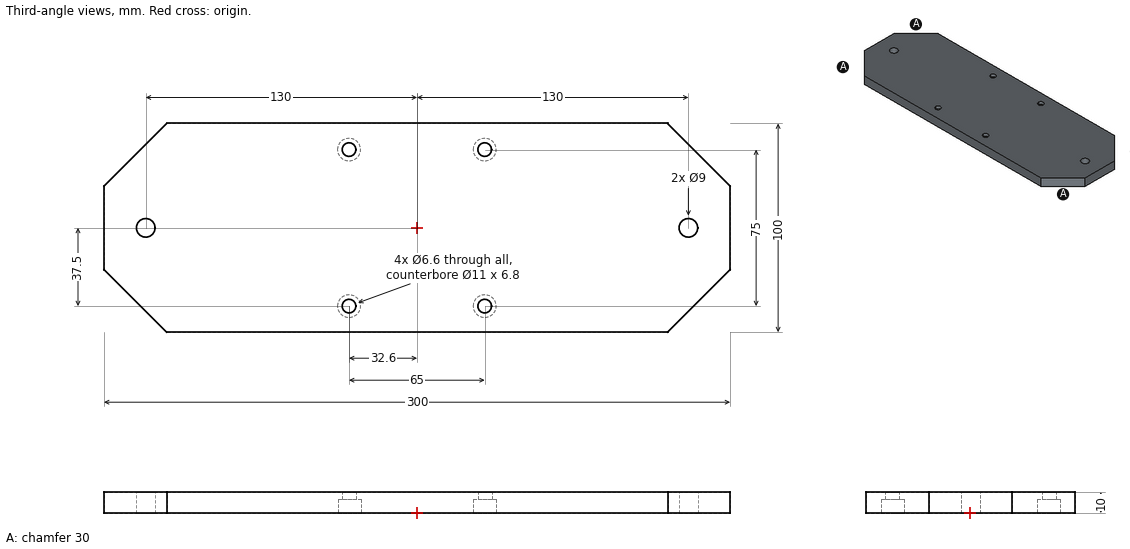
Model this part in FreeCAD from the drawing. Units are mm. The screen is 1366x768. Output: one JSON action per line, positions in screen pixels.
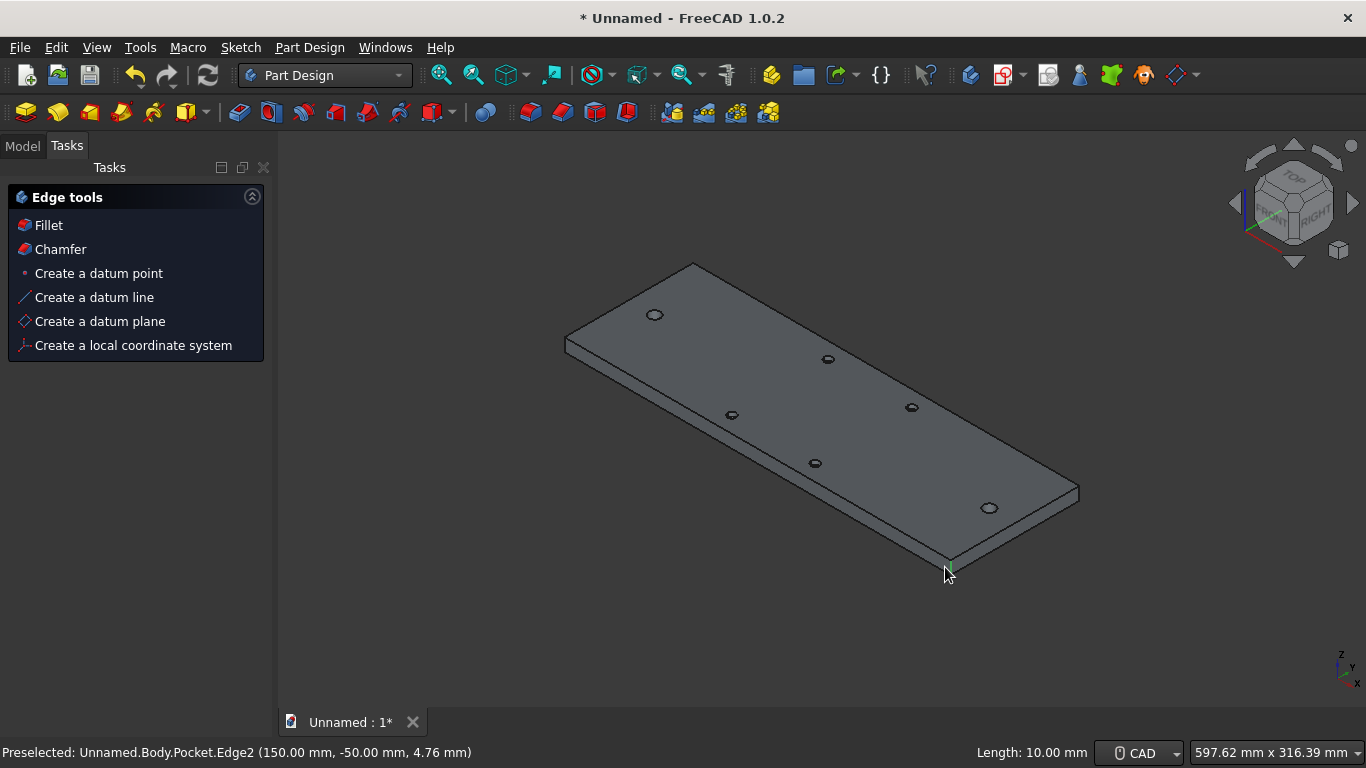
{"action": "scroll", "coordinate": [693, 269], "scroll_direction": "up", "scroll_amount": 4}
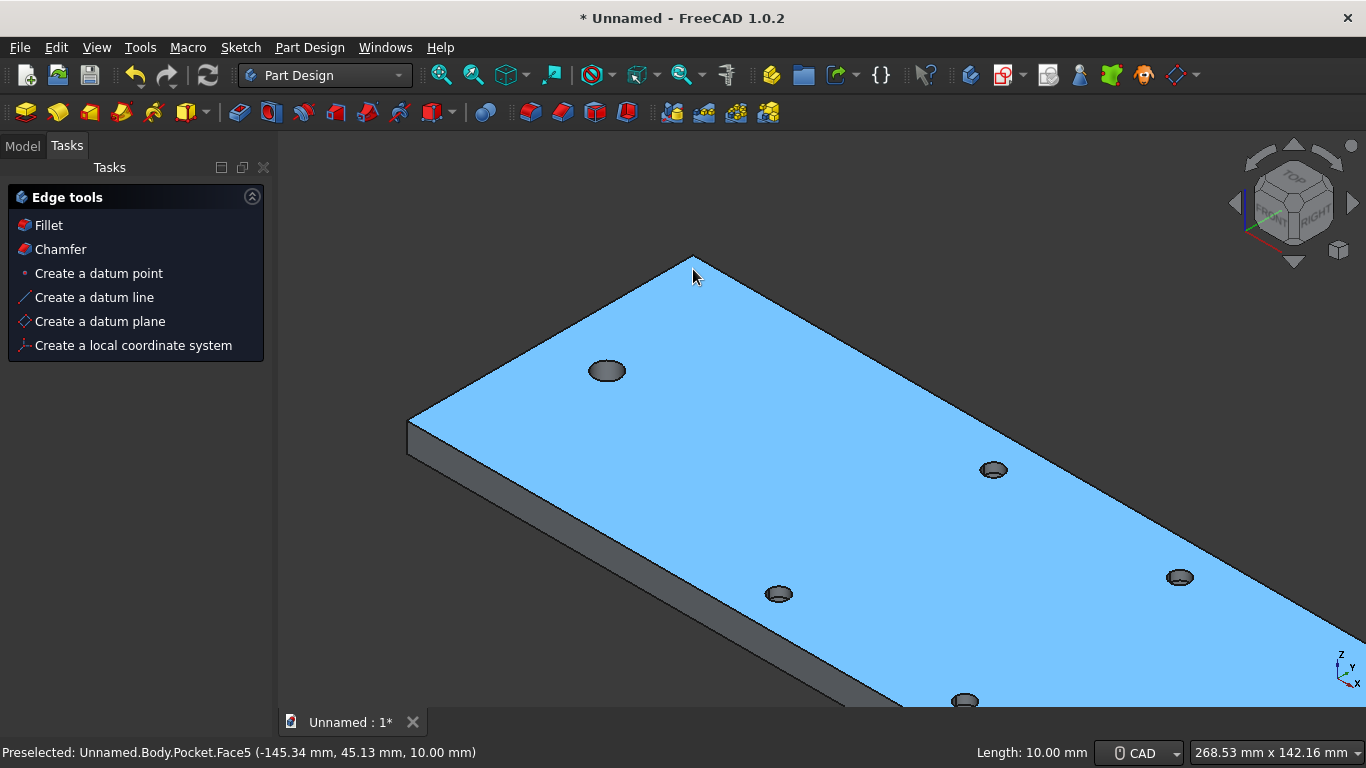
{"action": "left_click", "coordinate": [442, 76]}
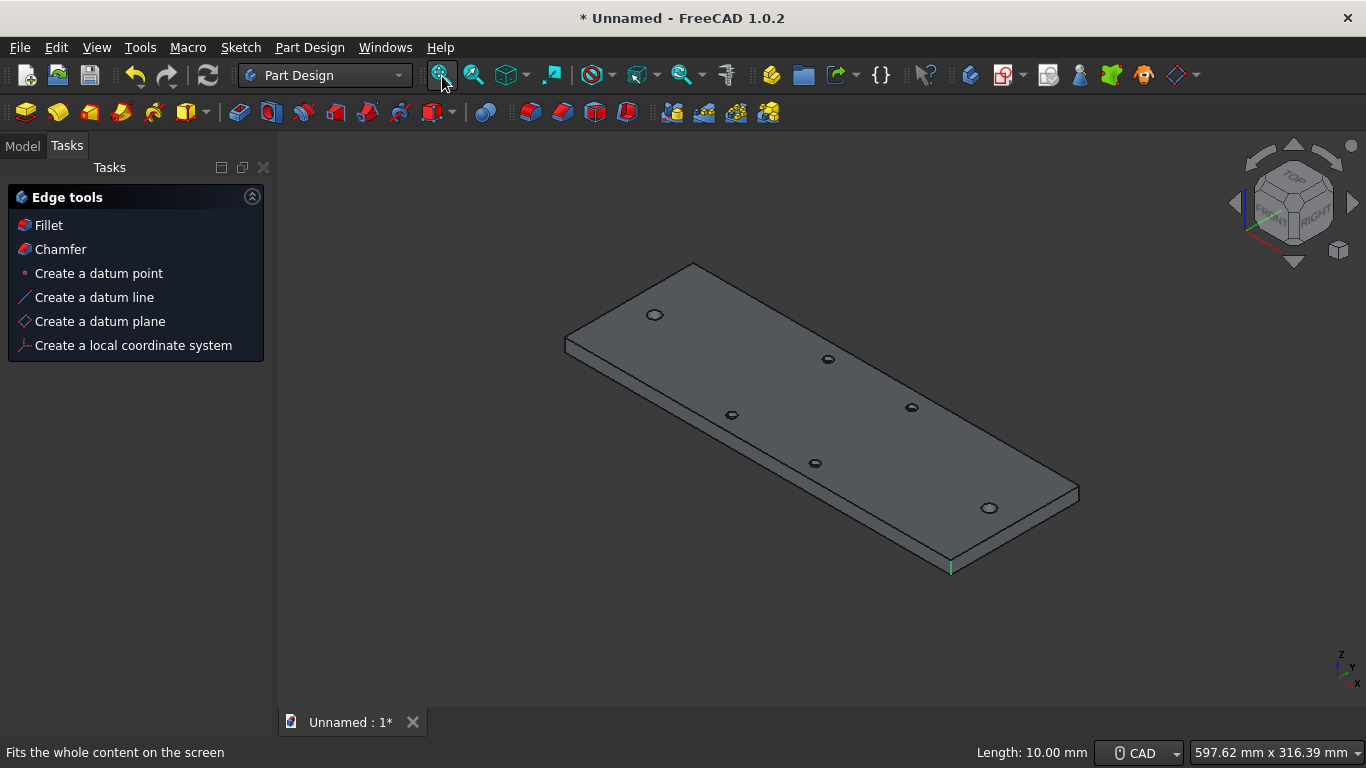
{"action": "key", "text": "2"}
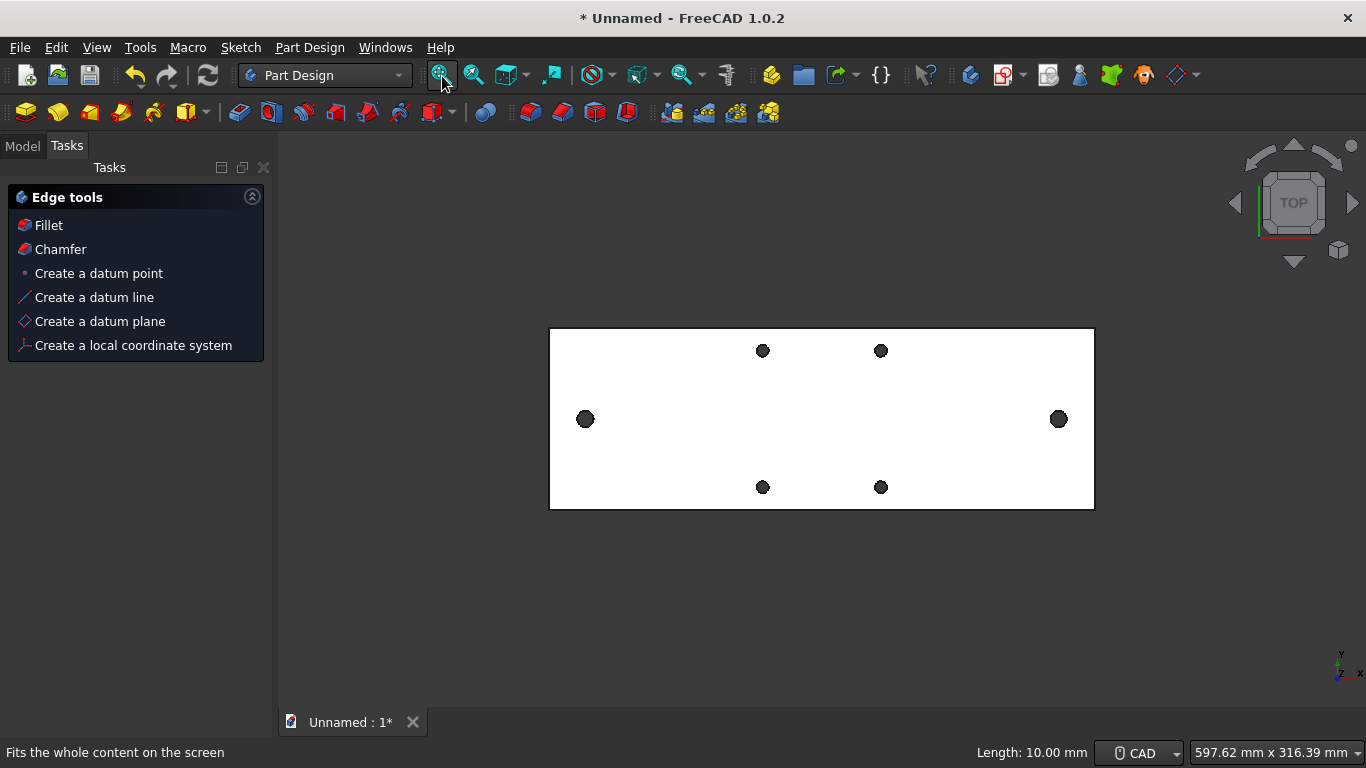
{"action": "scroll", "coordinate": [549, 327], "scroll_direction": "up", "scroll_amount": 4}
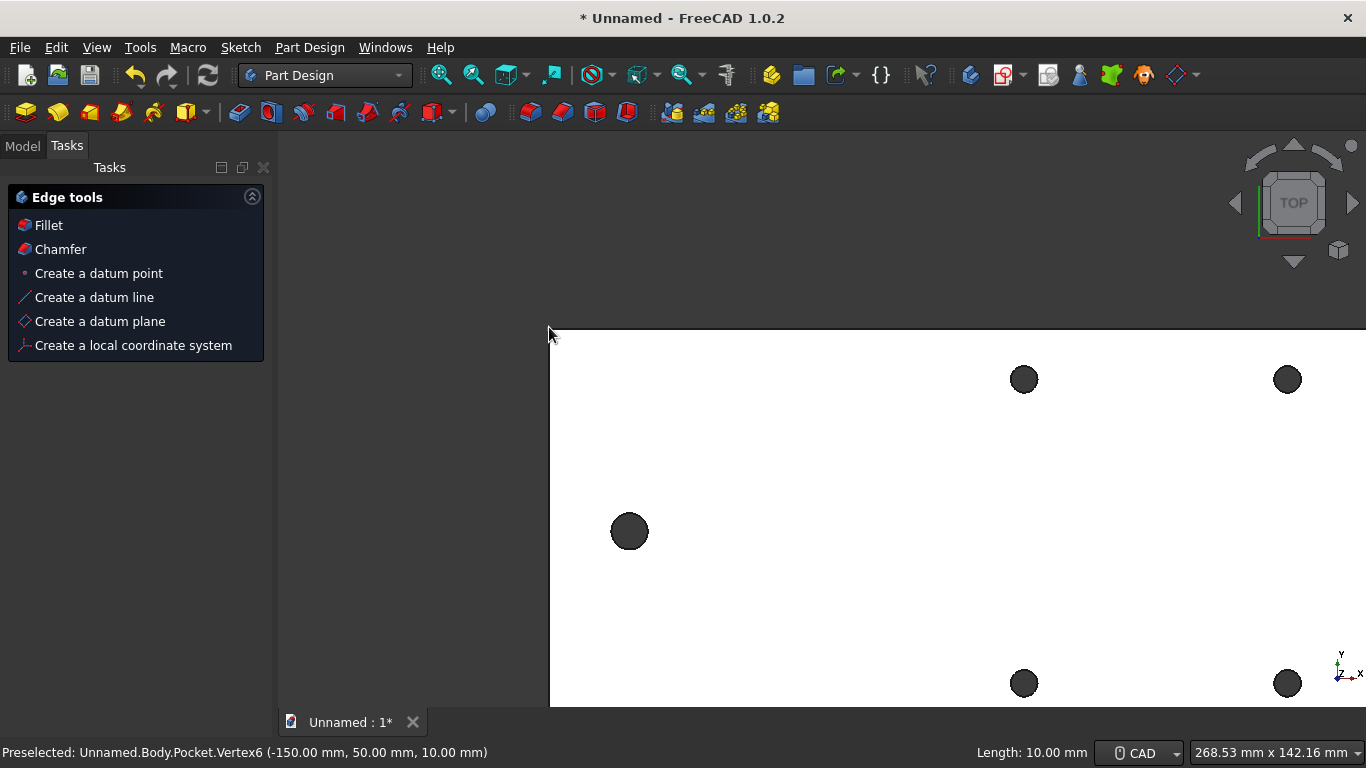
{"action": "key", "text": "v f"}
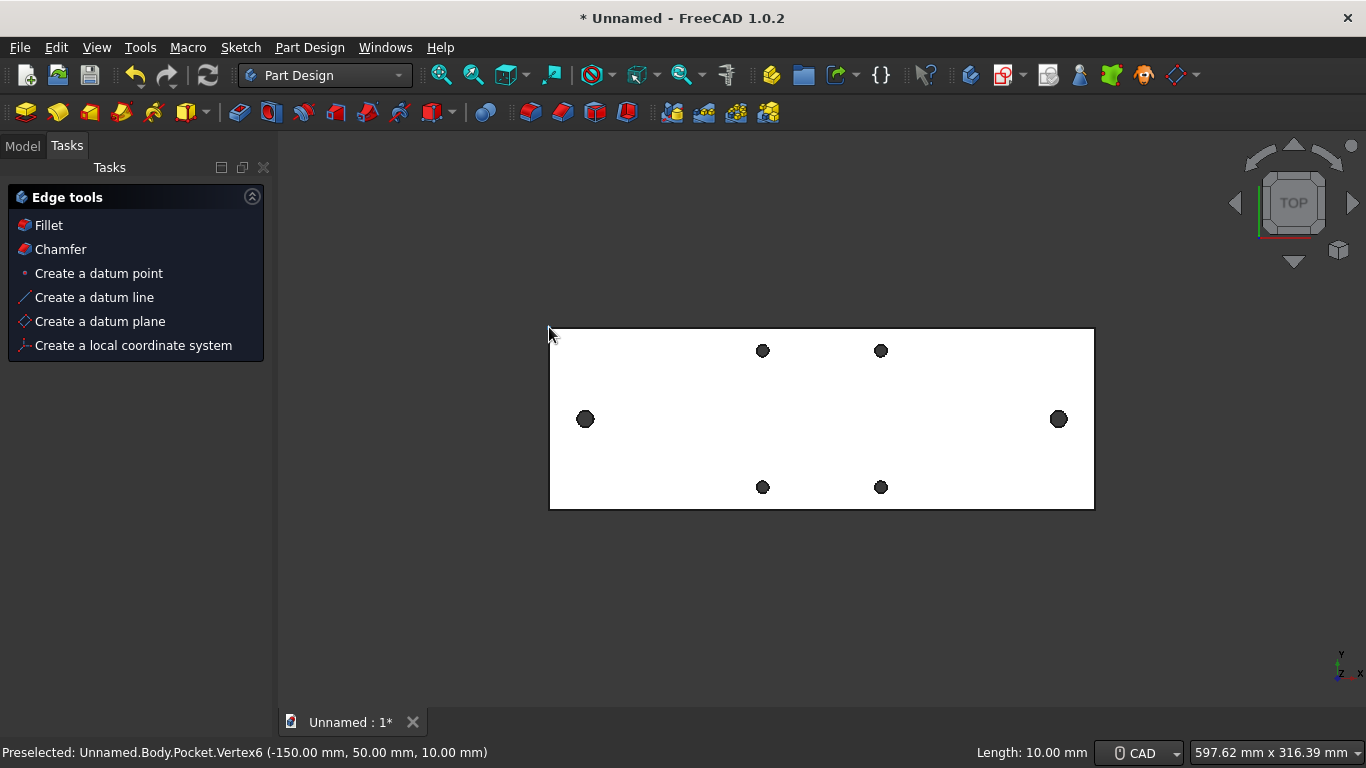
{"action": "key", "text": "1"}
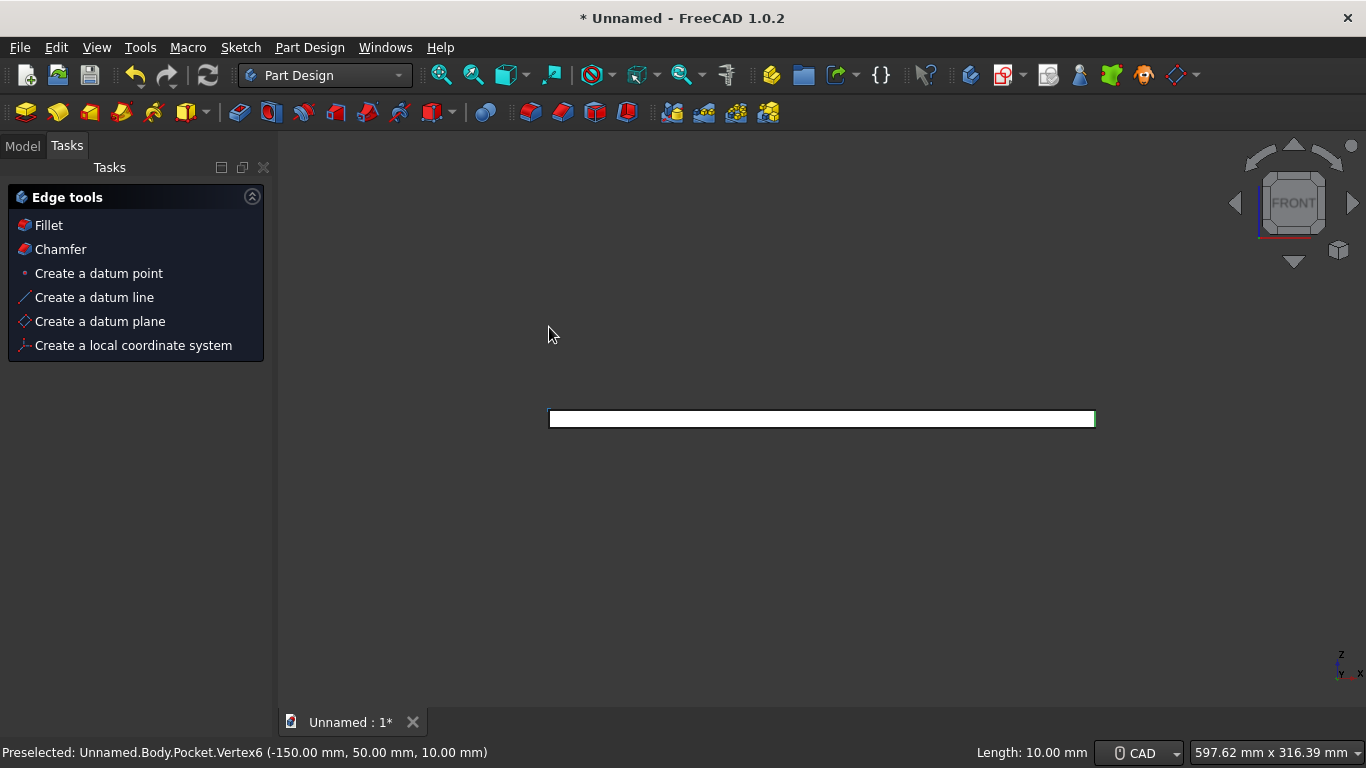
{"action": "left_click", "coordinate": [549, 418], "text": "ctrl"}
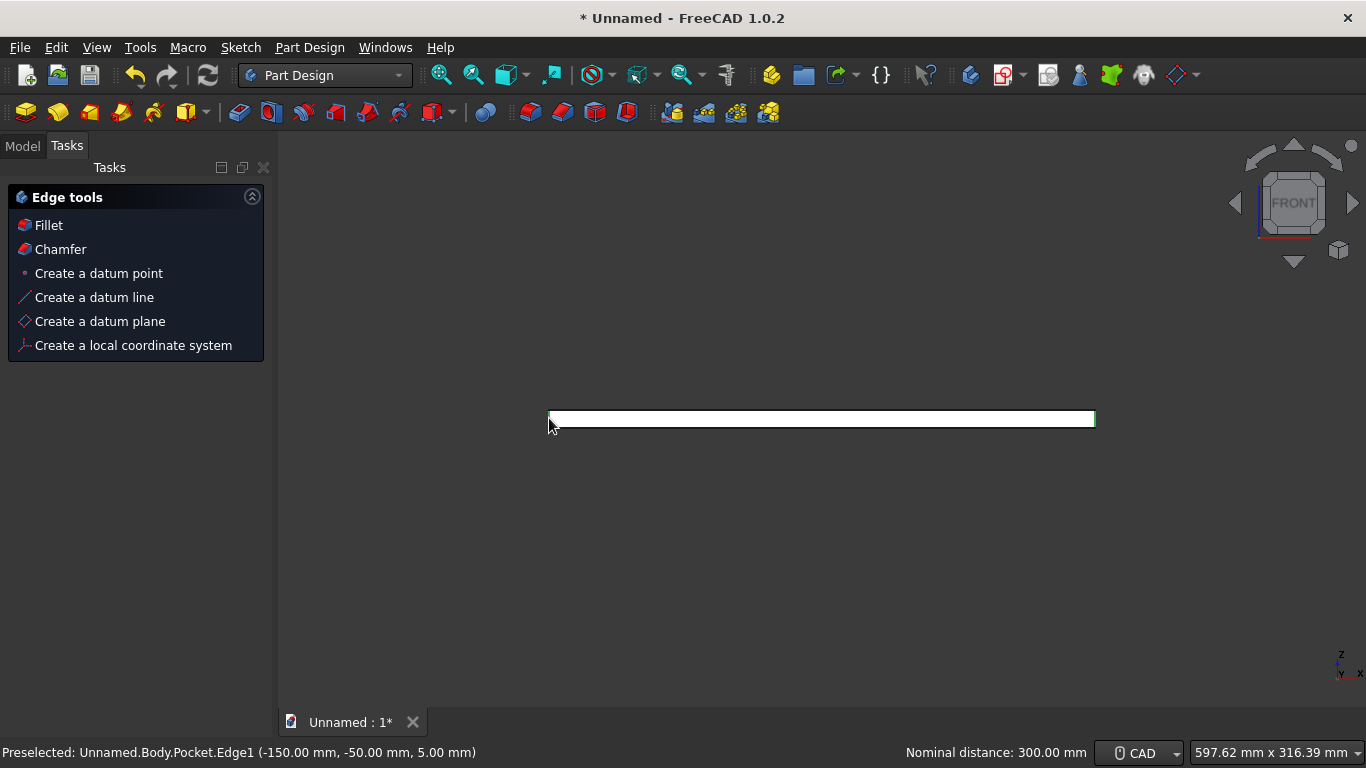
{"action": "scroll", "coordinate": [549, 418], "scroll_direction": "up", "scroll_amount": 4}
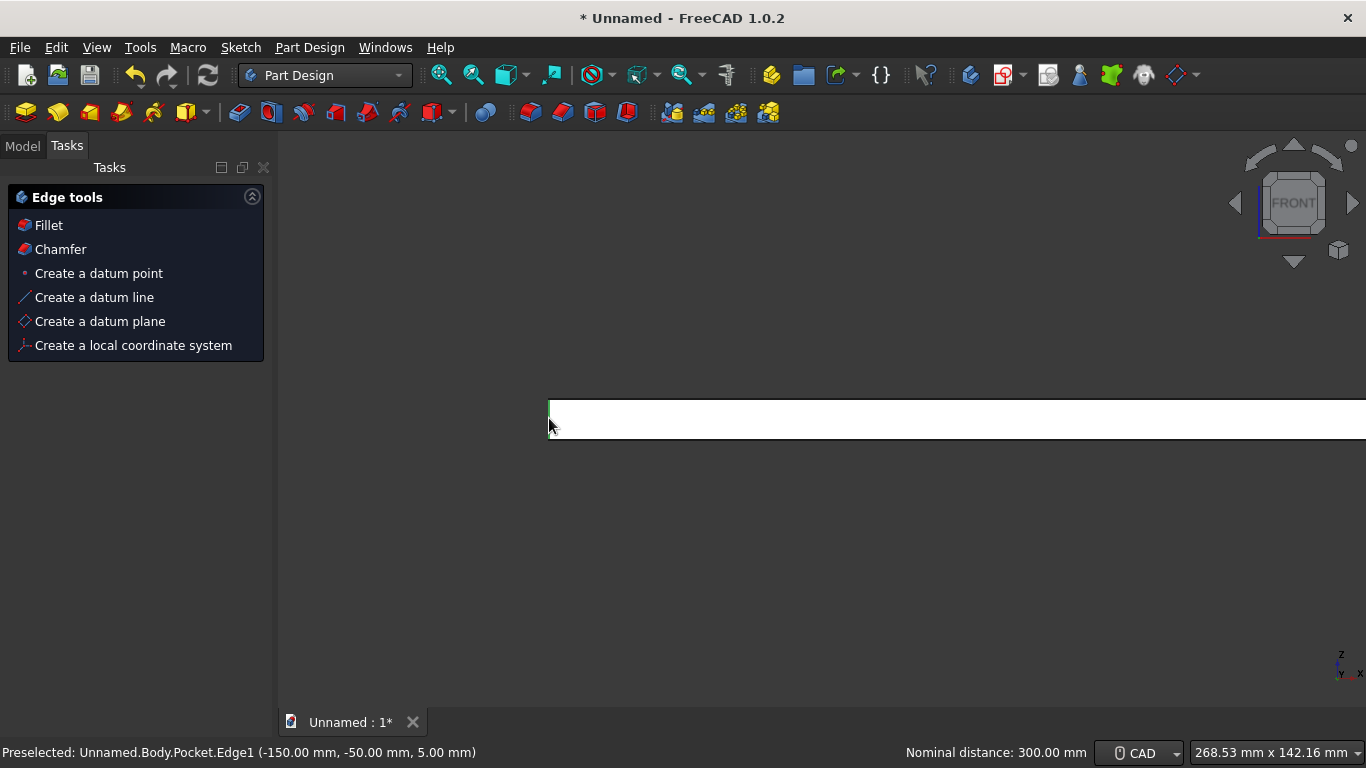
{"action": "left_click", "coordinate": [442, 76]}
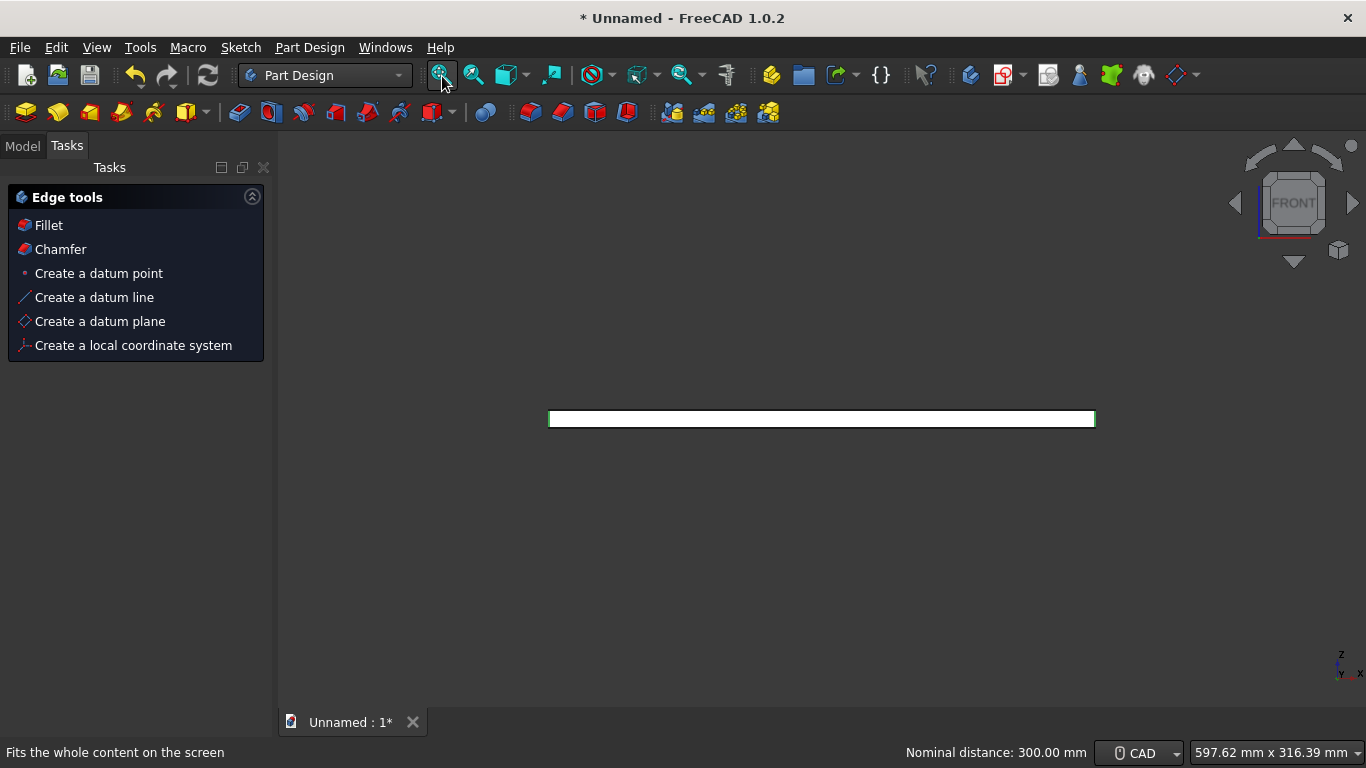
{"action": "key", "text": "3"}